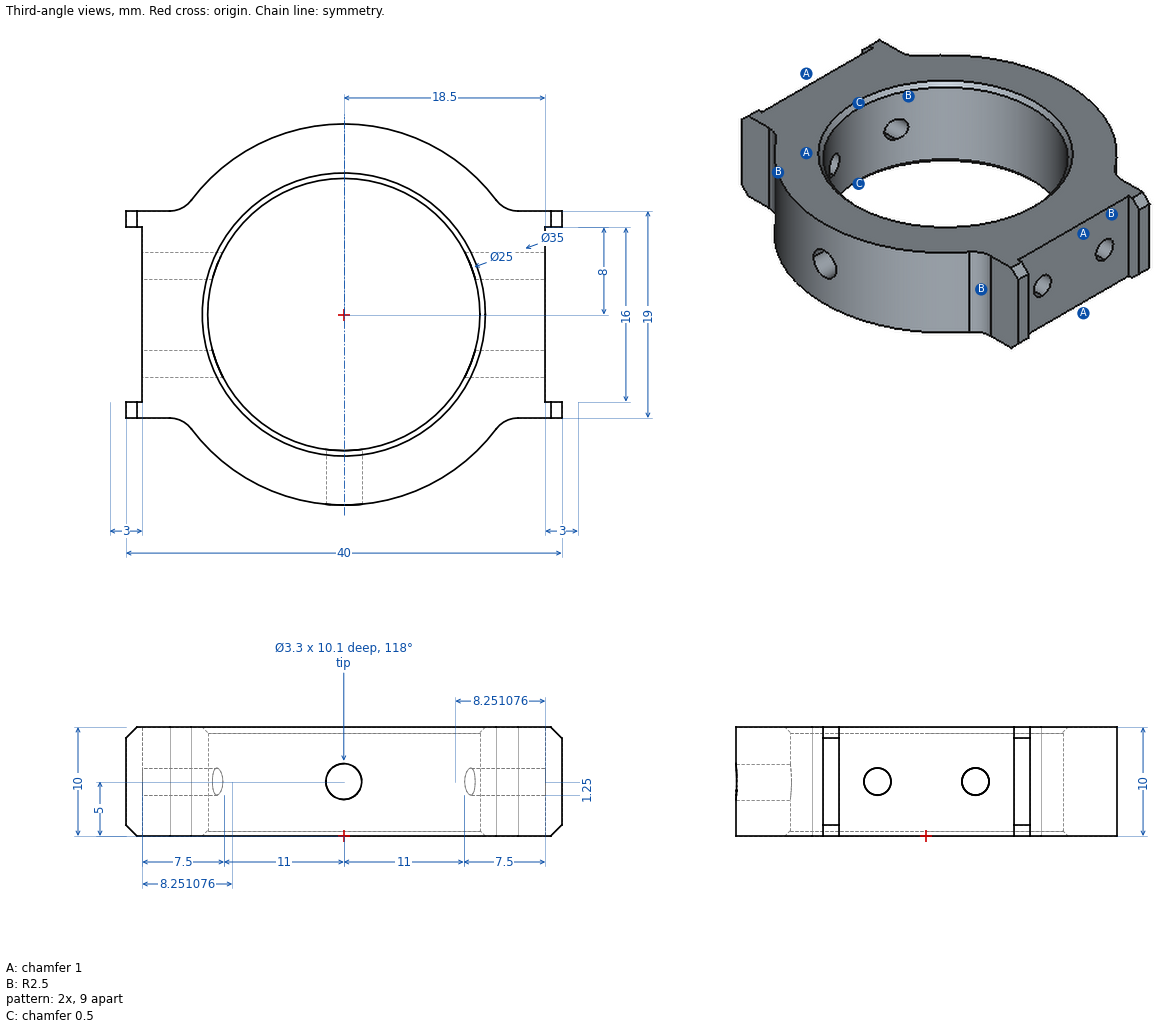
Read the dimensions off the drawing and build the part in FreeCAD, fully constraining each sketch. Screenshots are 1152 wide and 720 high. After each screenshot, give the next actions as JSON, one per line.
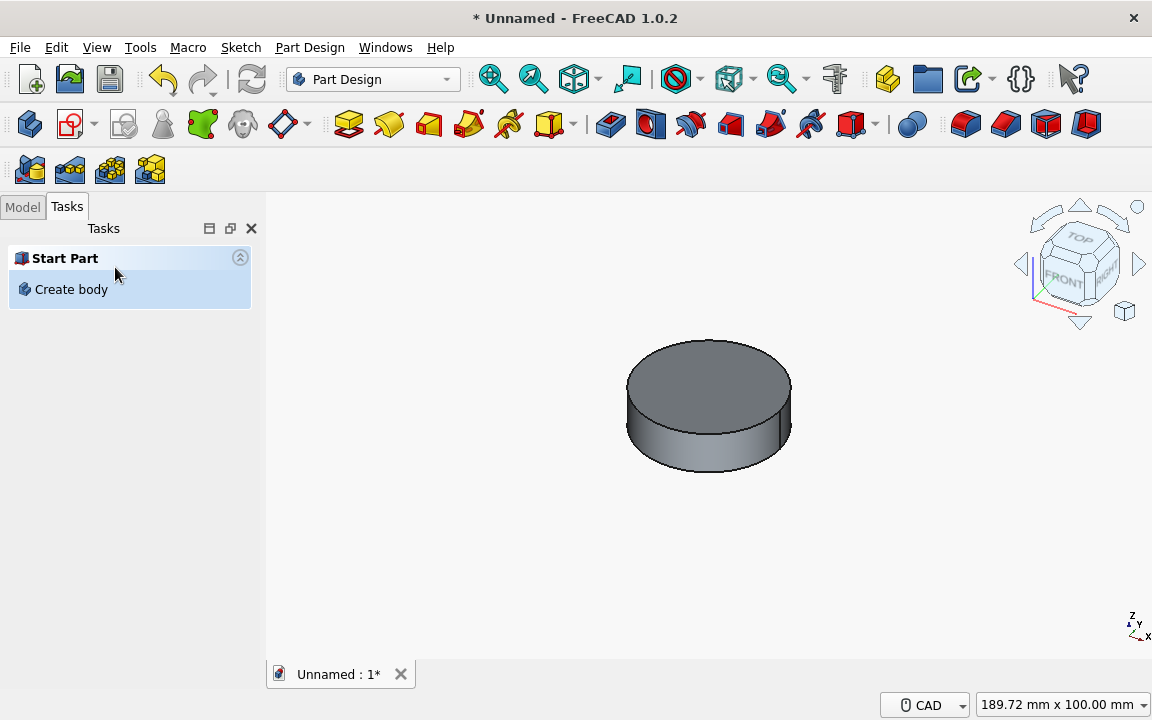
{"action": "left_click", "coordinate": [494, 80]}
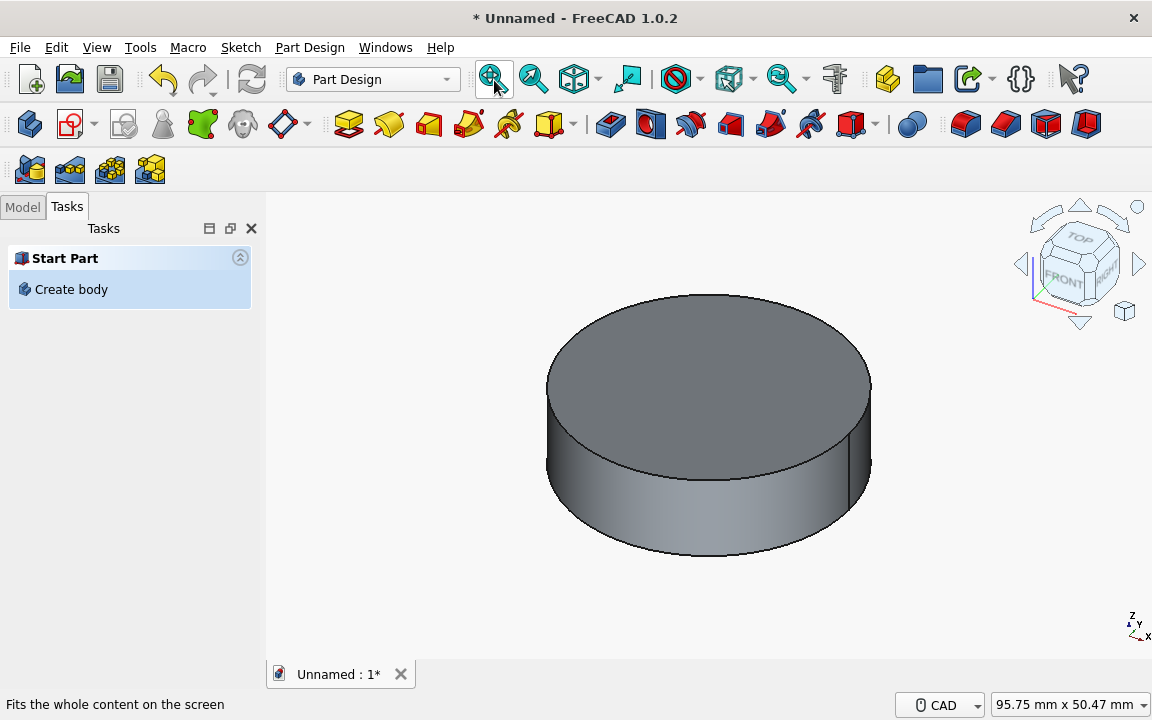
{"action": "left_click", "coordinate": [709, 387]}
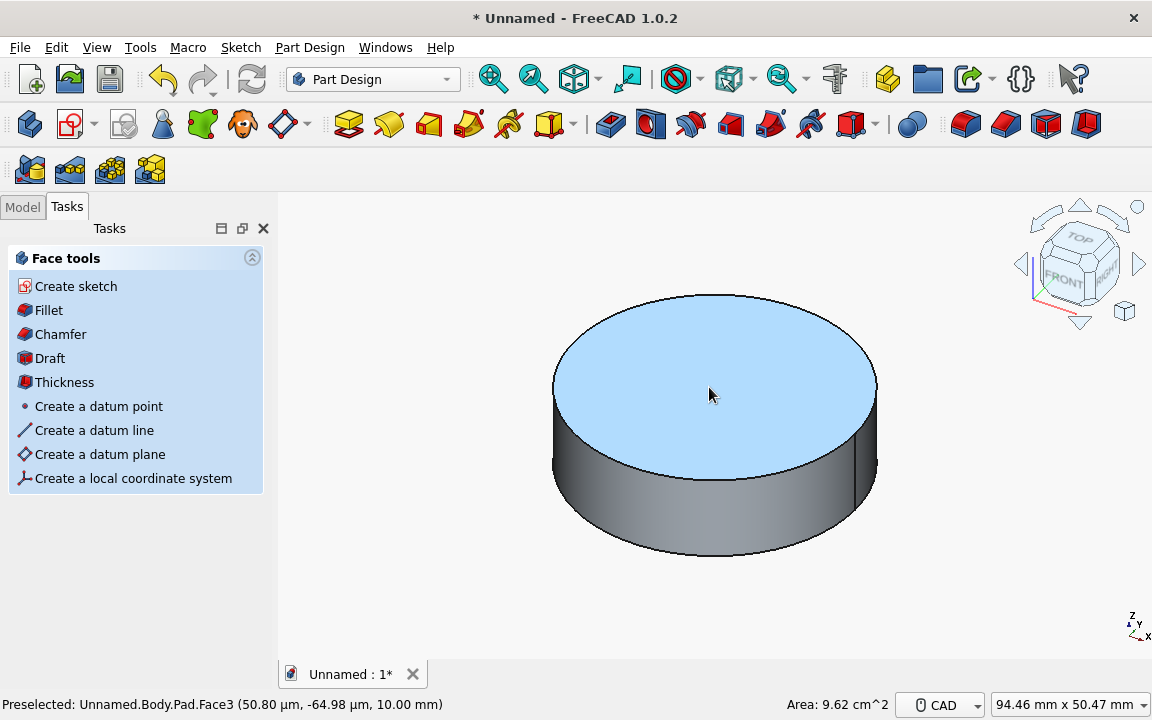
{"action": "left_click", "coordinate": [70, 124]}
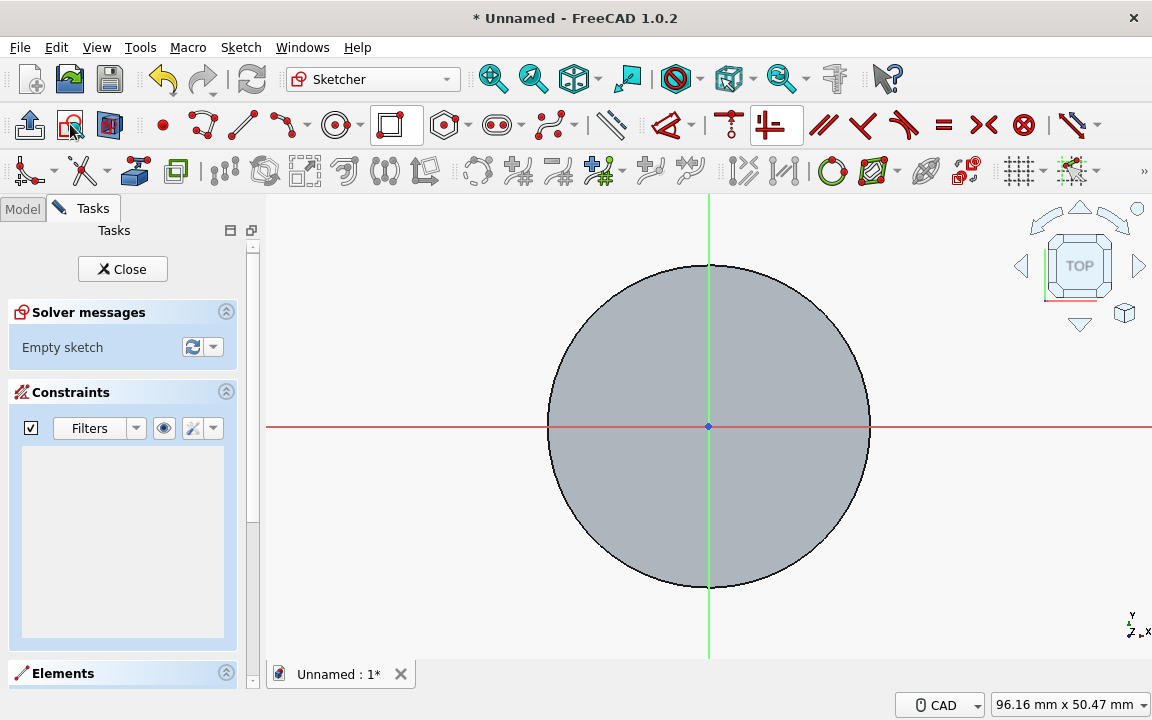
{"action": "left_click", "coordinate": [418, 126]}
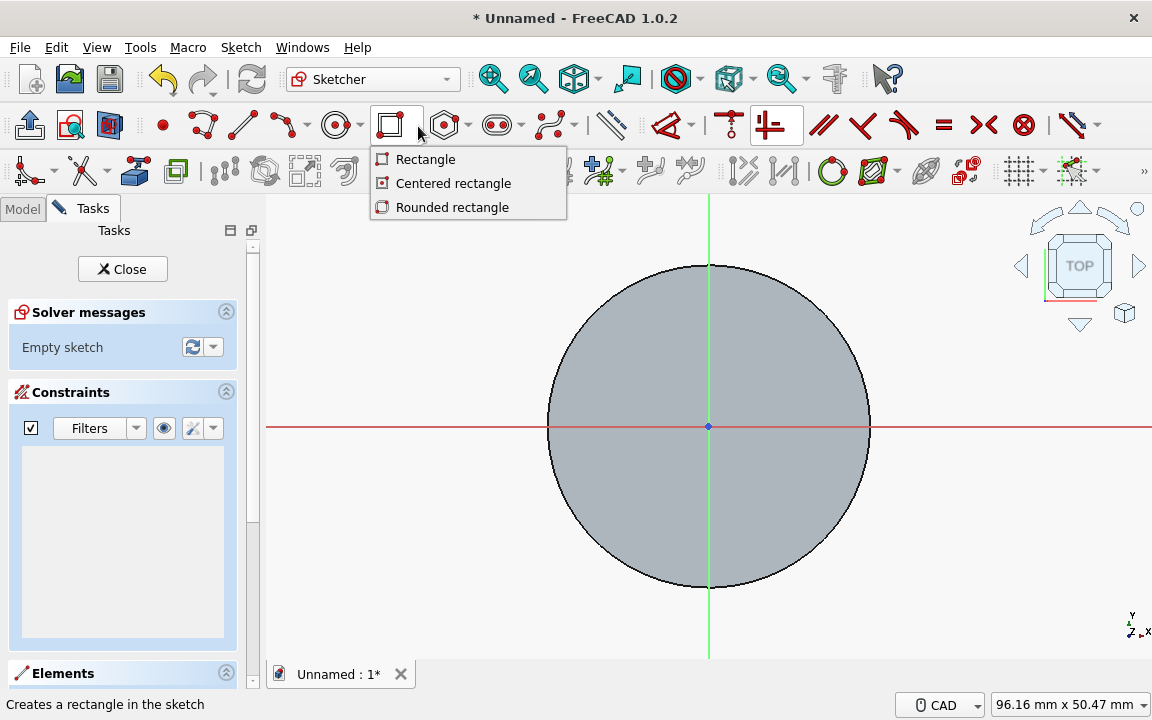
{"action": "left_click", "coordinate": [468, 183]}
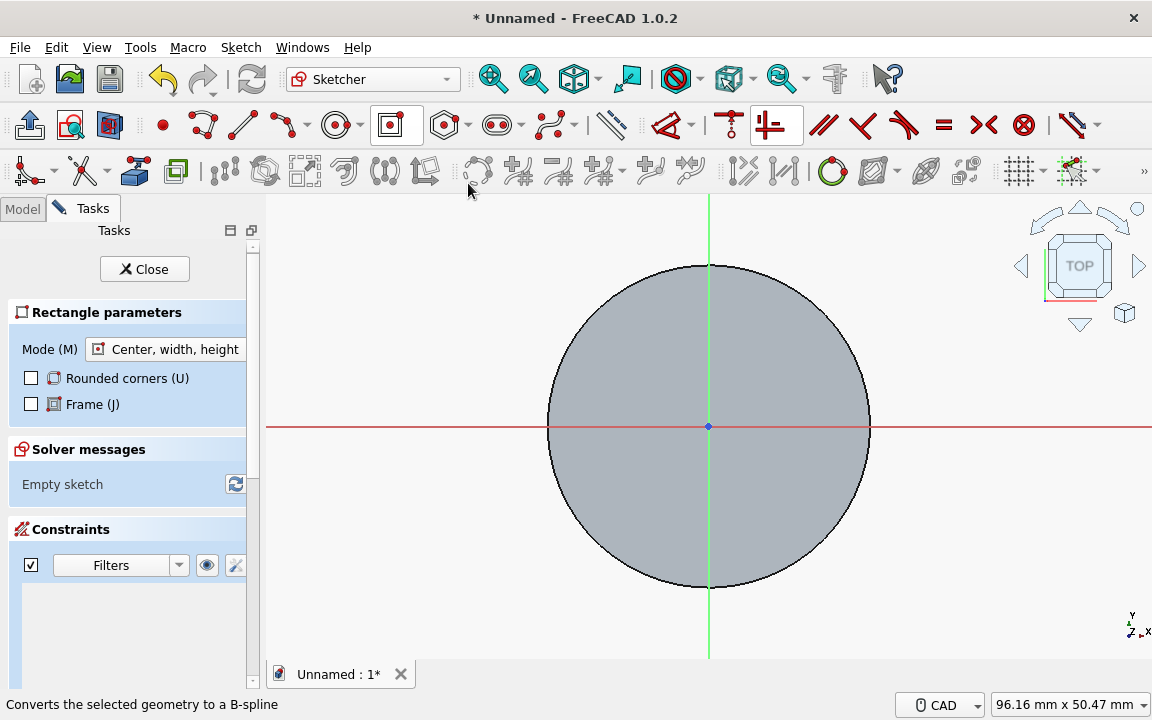
{"action": "left_click", "coordinate": [709, 426]}
{"action": "mouse_move", "coordinate": [893, 339]}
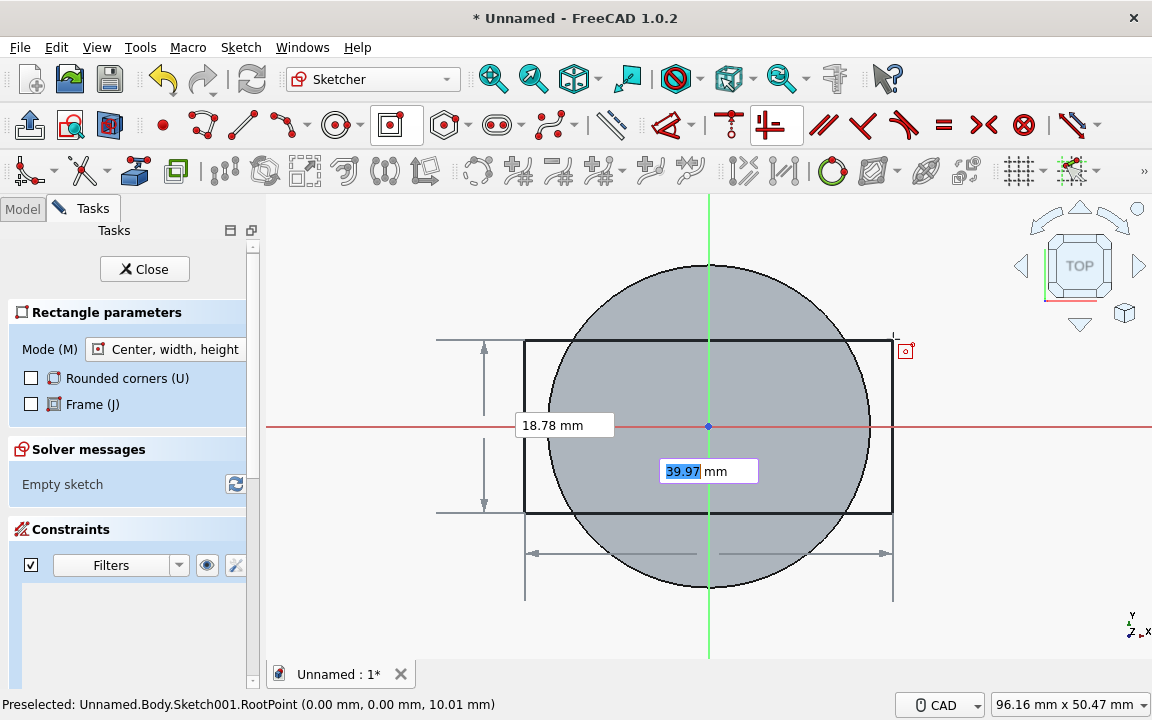
{"action": "type", "text": "40"}
{"action": "key", "text": "Tab"}
{"action": "type", "text": "19"}
{"action": "key", "text": "Return"}
{"action": "key", "text": "Escape"}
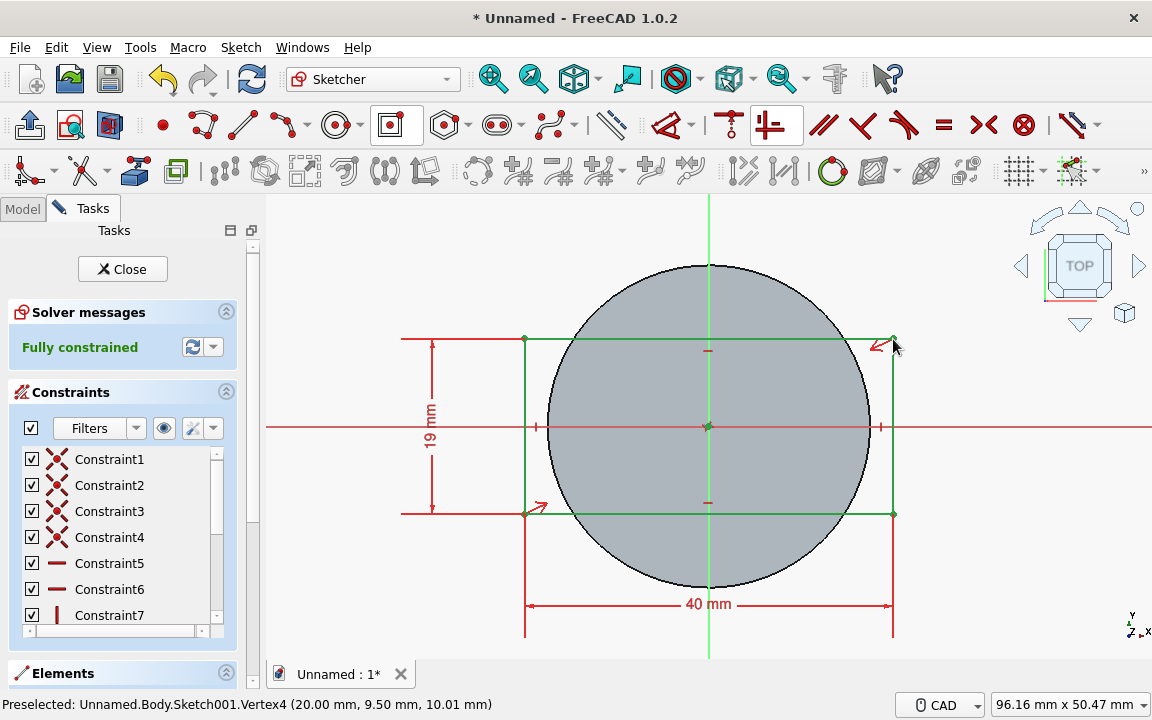
{"action": "left_click", "coordinate": [123, 269]}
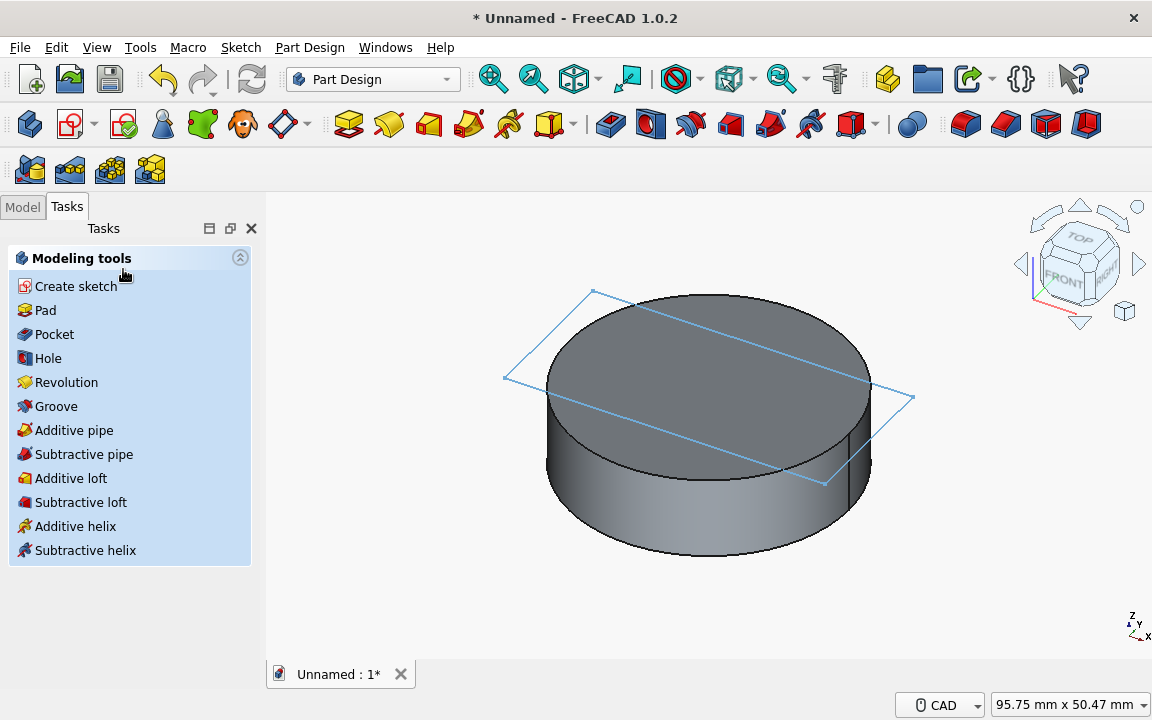
{"action": "left_click", "coordinate": [350, 124]}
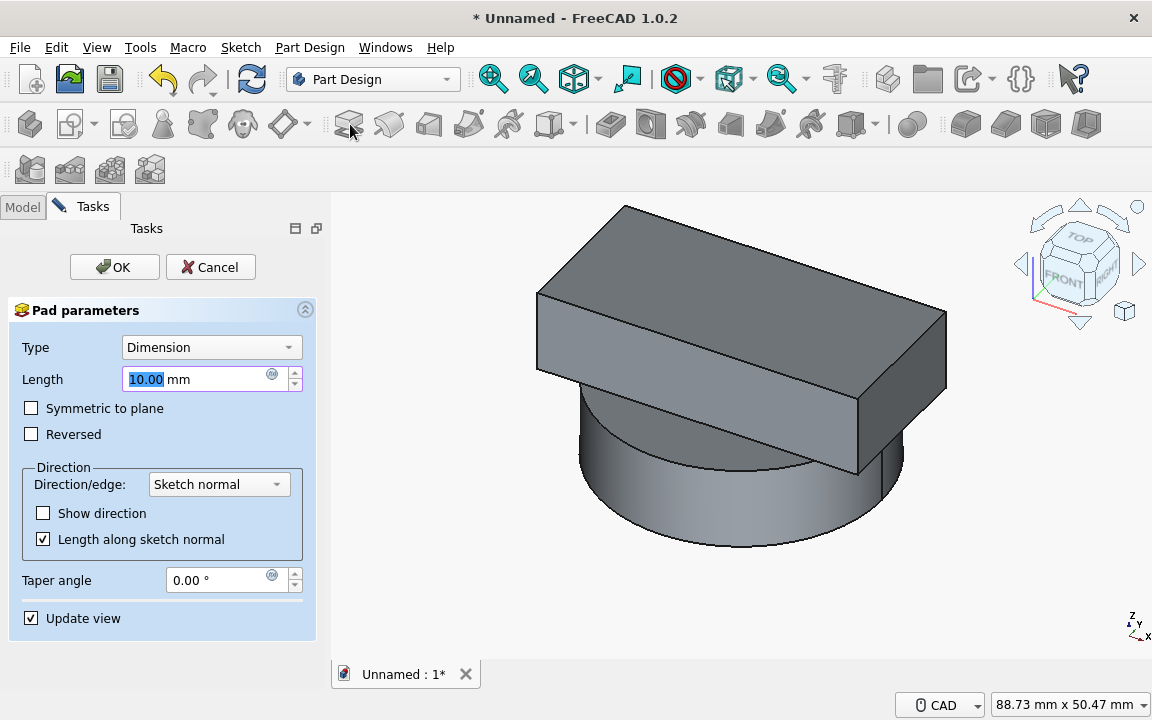
{"action": "type", "text": "10"}
{"action": "key", "text": "Tab"}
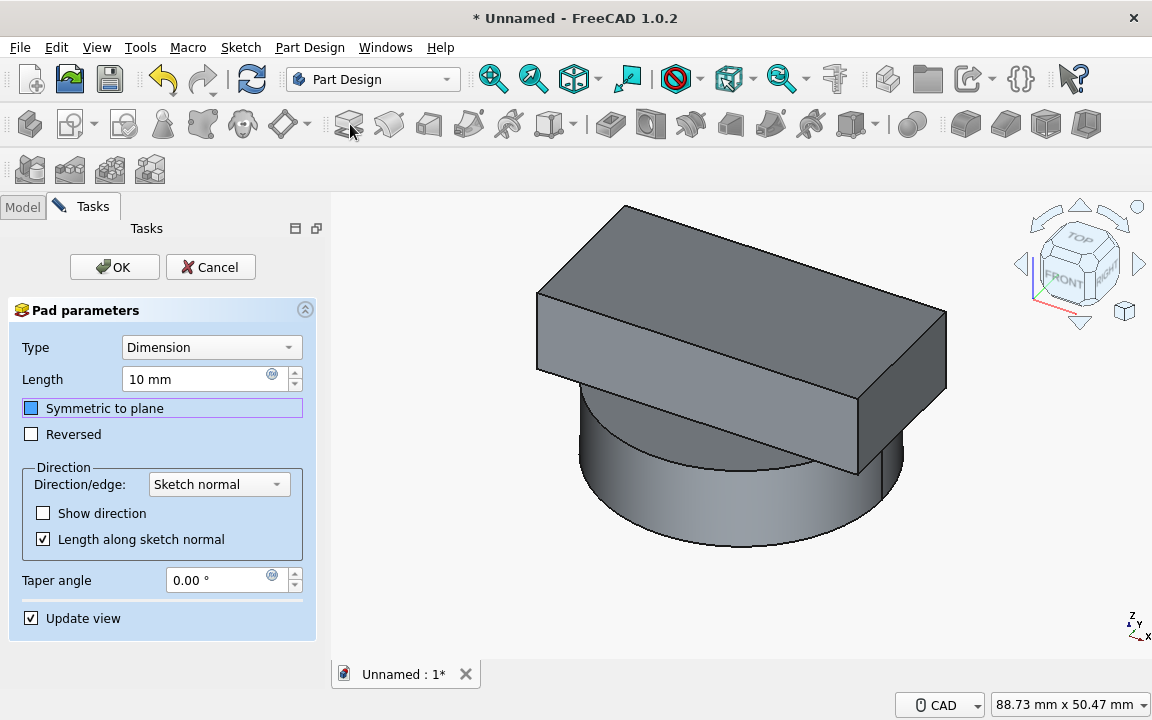
{"action": "left_click", "coordinate": [30, 434]}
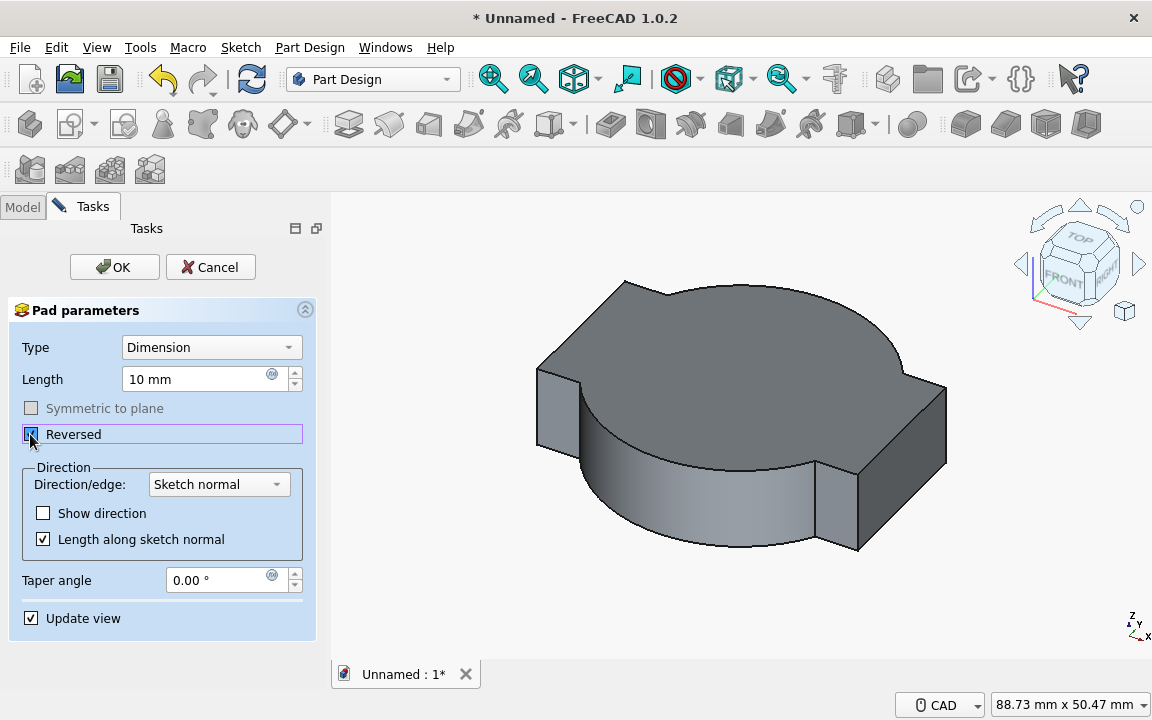
{"action": "left_click", "coordinate": [115, 267]}